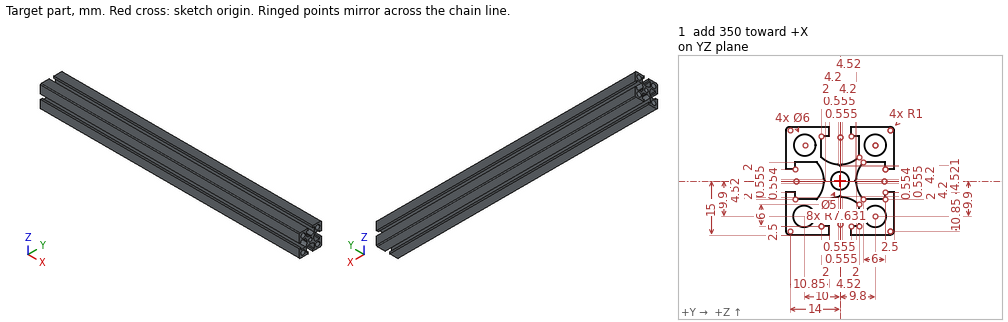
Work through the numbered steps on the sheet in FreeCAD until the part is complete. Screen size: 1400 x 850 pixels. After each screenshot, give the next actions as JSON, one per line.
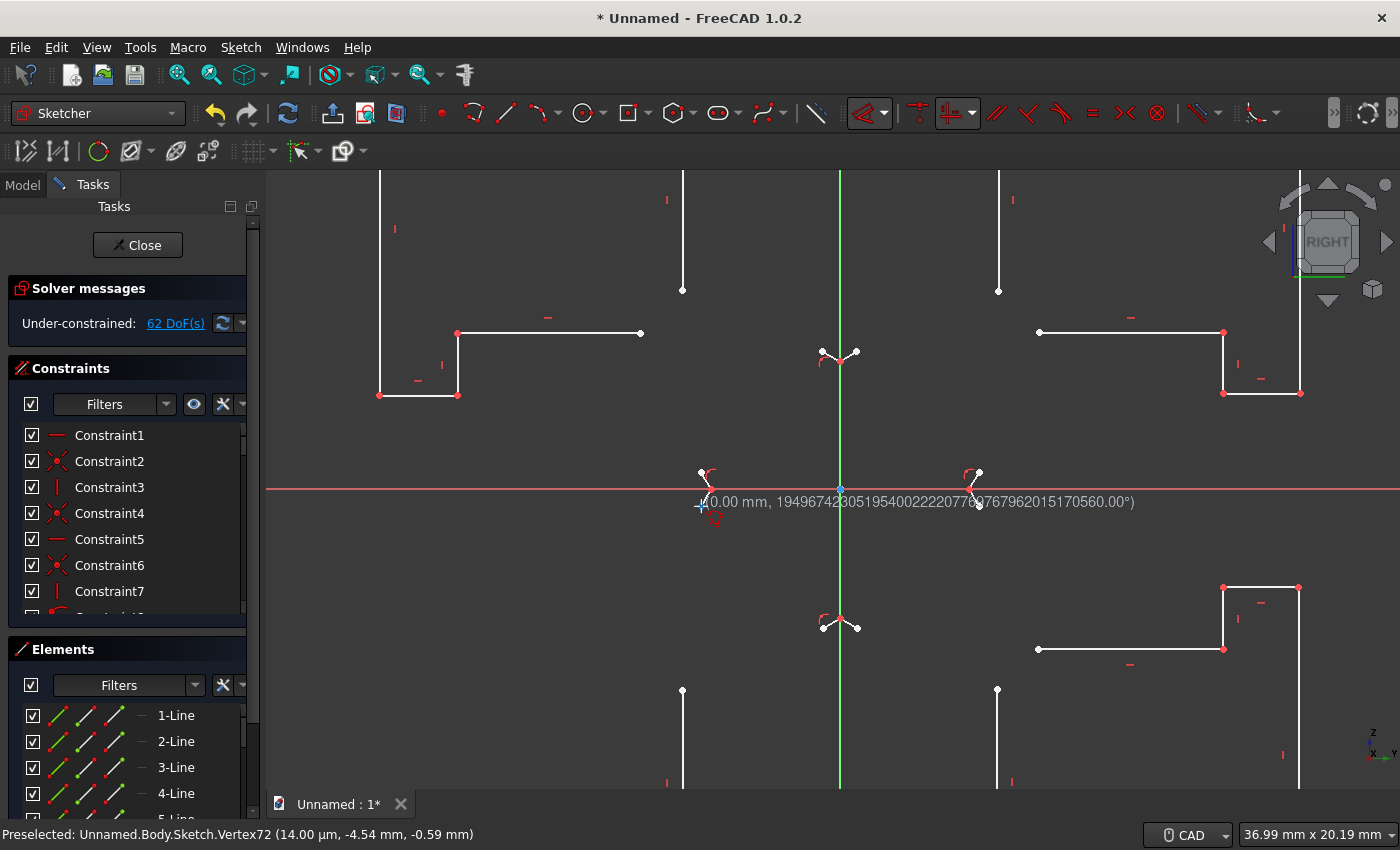
{"action": "left_click", "coordinate": [641, 647]}
{"action": "left_click", "coordinate": [457, 647]}
{"action": "left_click", "coordinate": [457, 586]}
{"action": "left_click", "coordinate": [380, 586]}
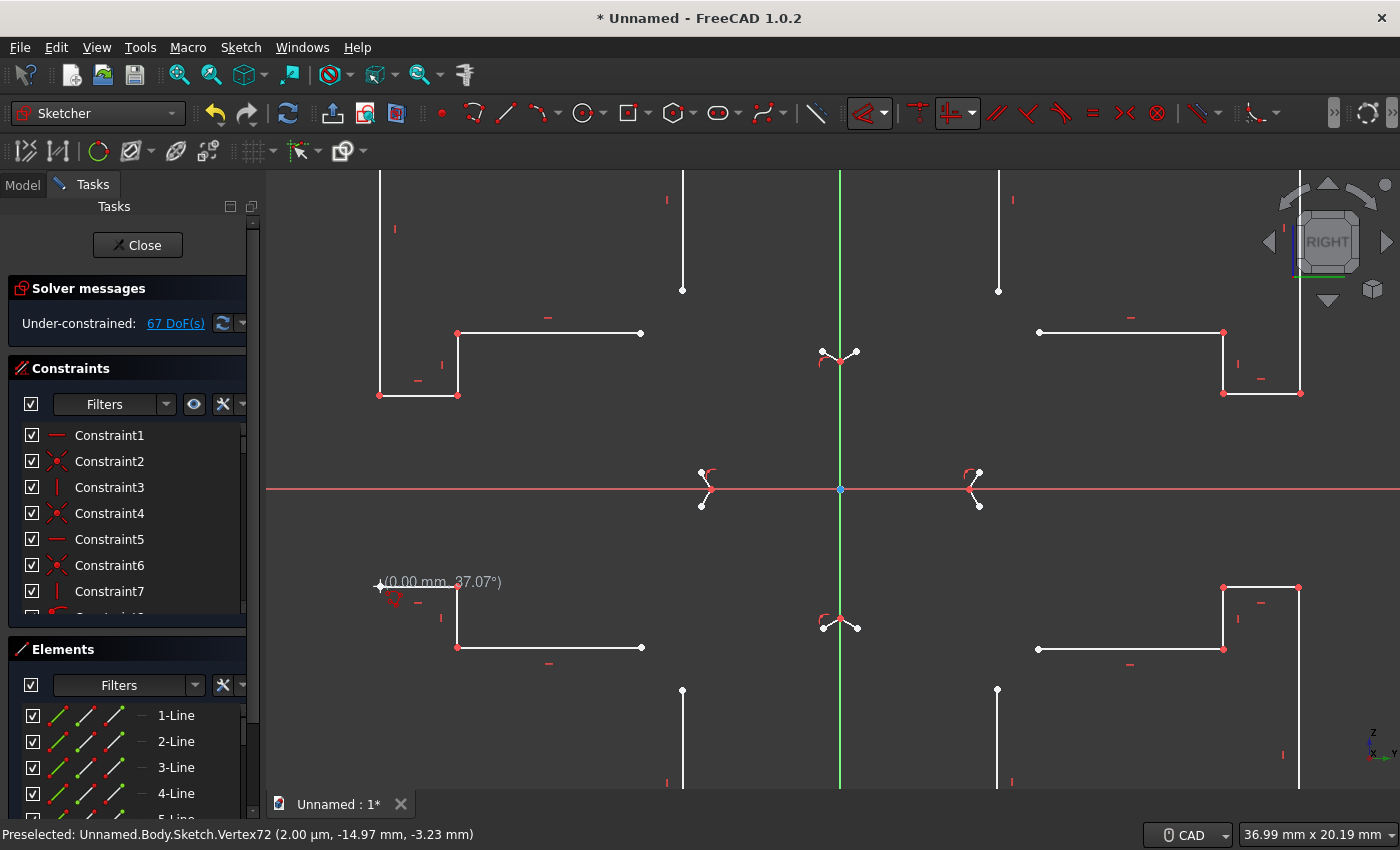
{"action": "scroll", "coordinate": [703, 472], "scroll_direction": "down", "scroll_amount": 4}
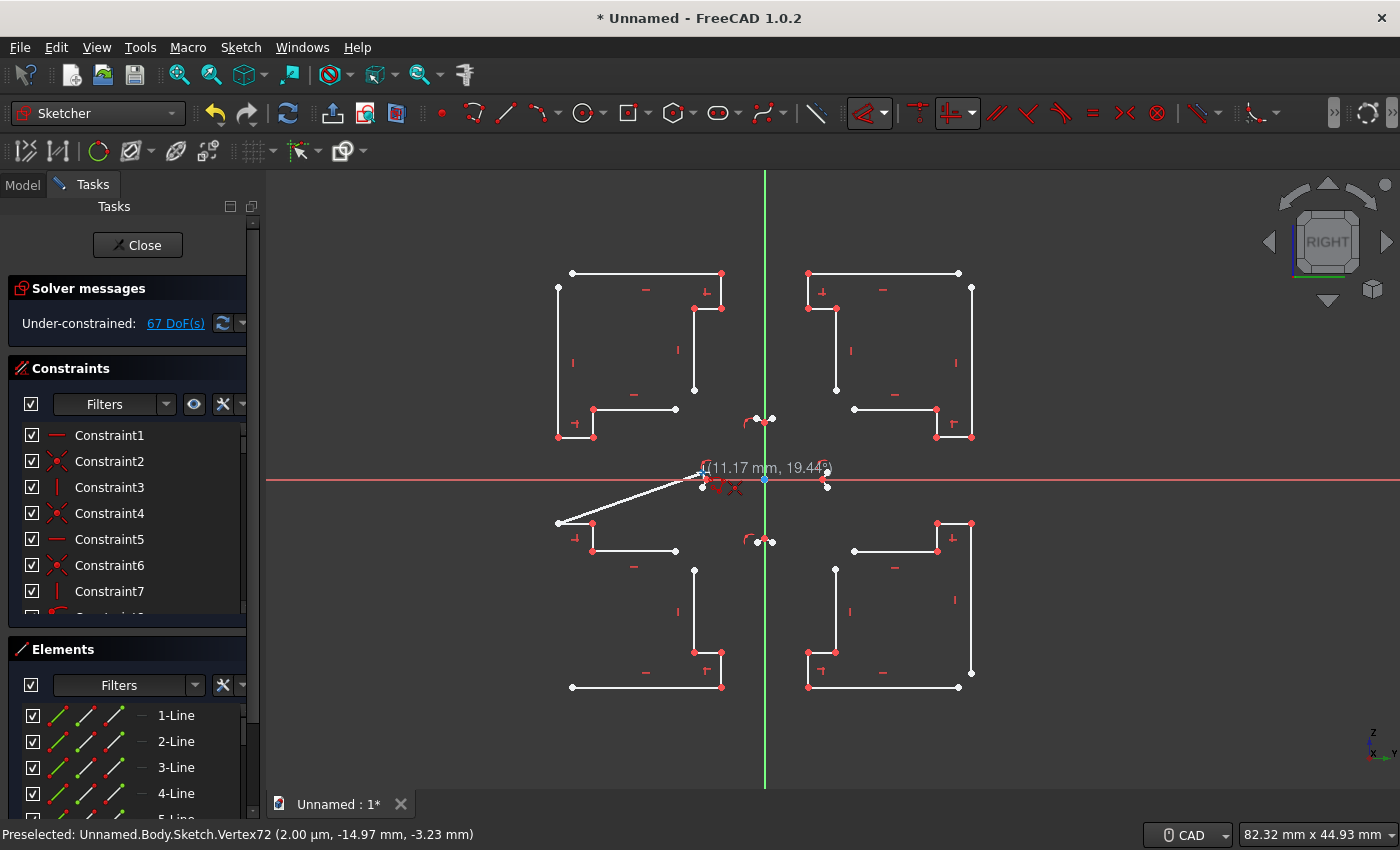
{"action": "left_click", "coordinate": [558, 673]}
{"action": "right_click", "coordinate": [558, 673]}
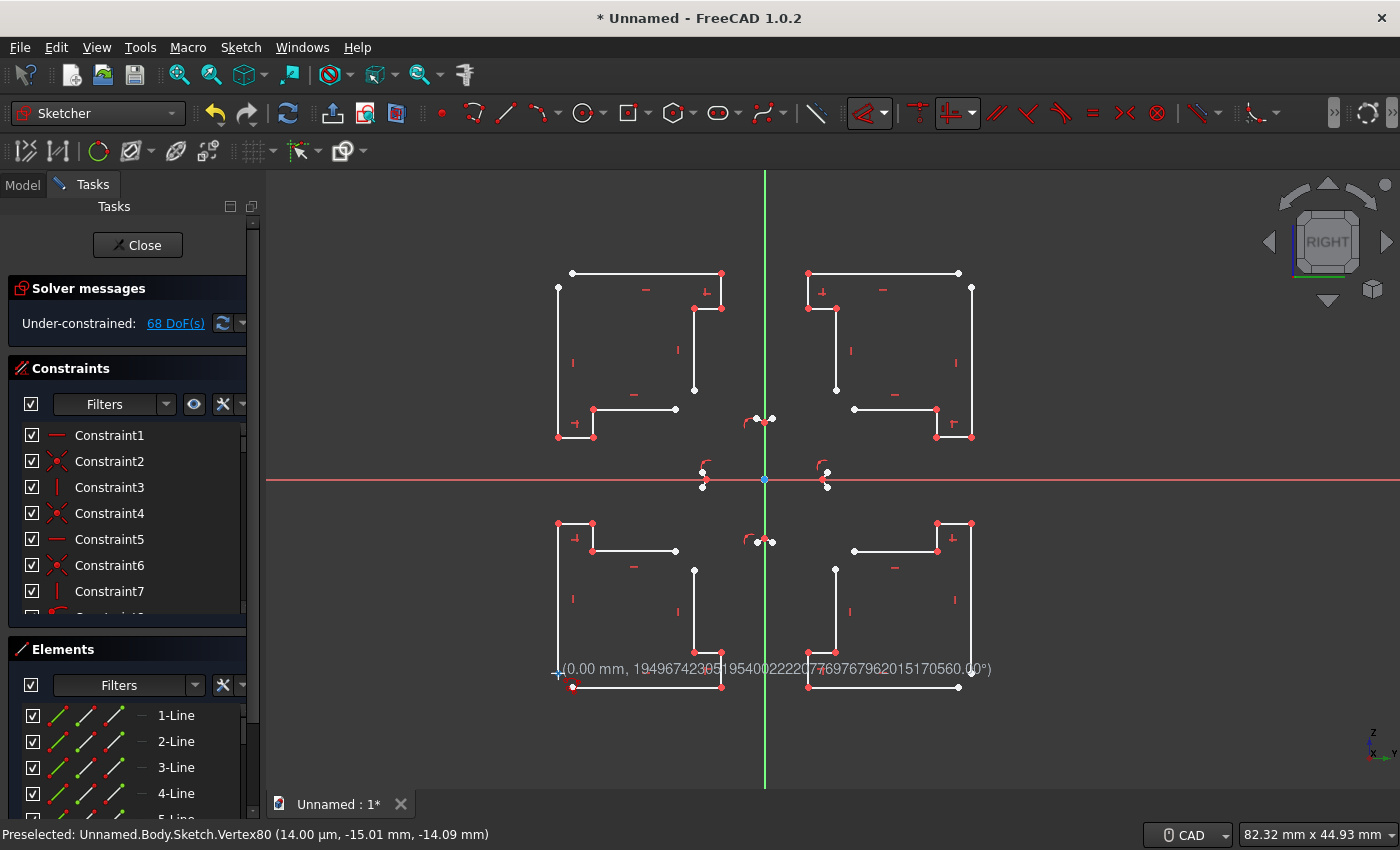
{"action": "left_click", "coordinate": [538, 114]}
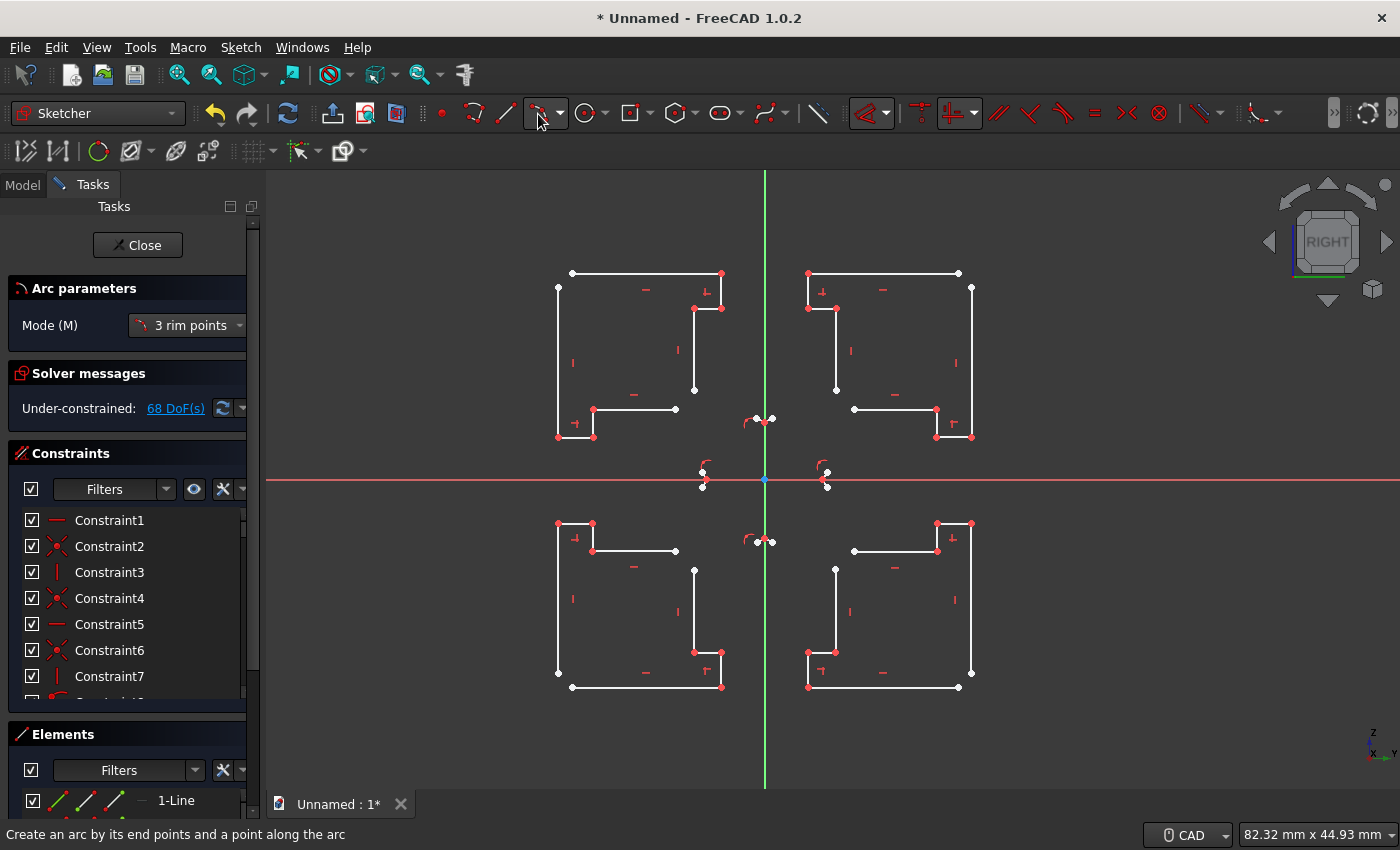
{"action": "left_click", "coordinate": [694, 571]}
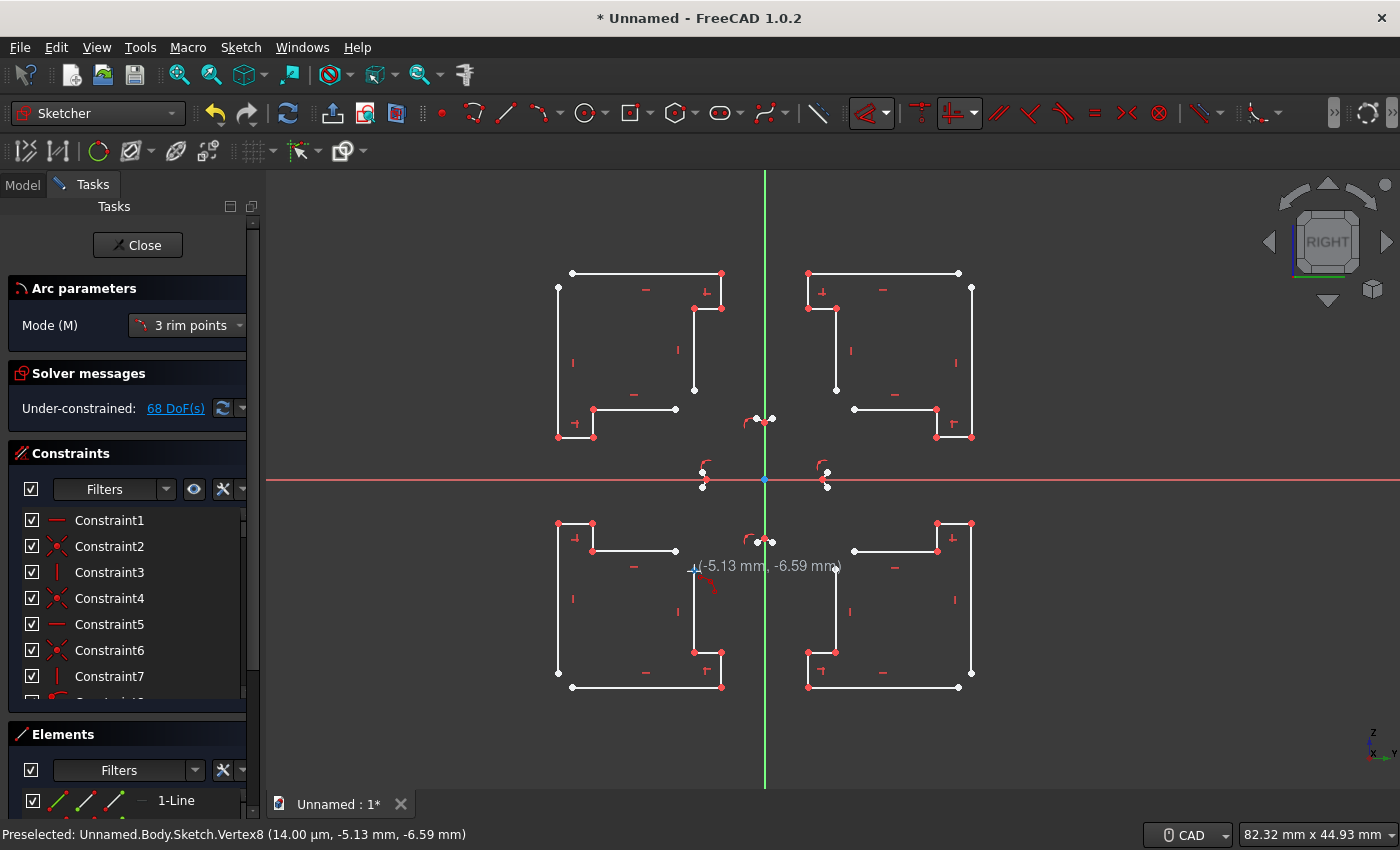
{"action": "scroll", "coordinate": [757, 542], "scroll_direction": "up", "scroll_amount": 7}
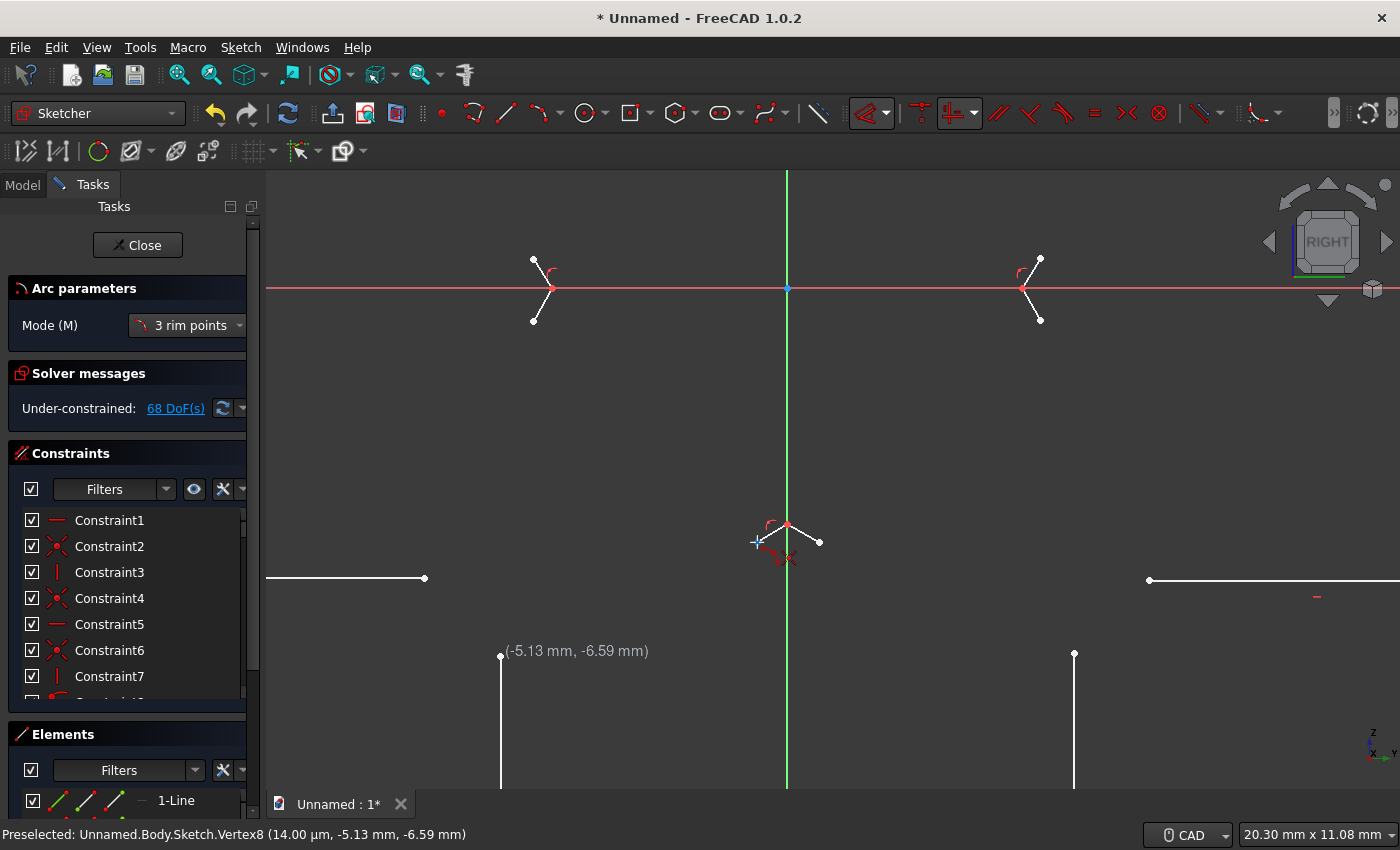
{"action": "left_click", "coordinate": [757, 542]}
{"action": "left_click", "coordinate": [619, 575]}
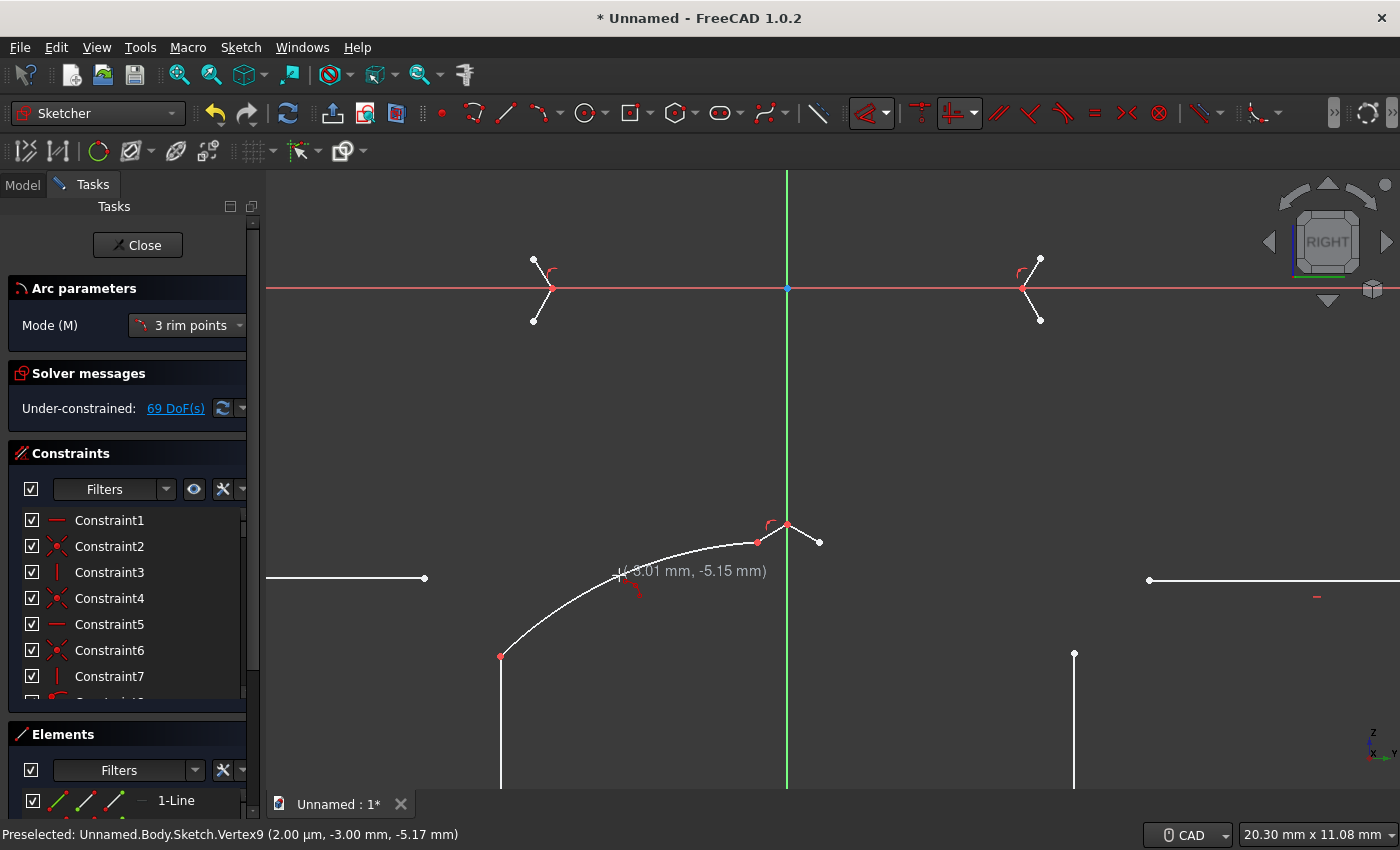
{"action": "left_click", "coordinate": [819, 542]}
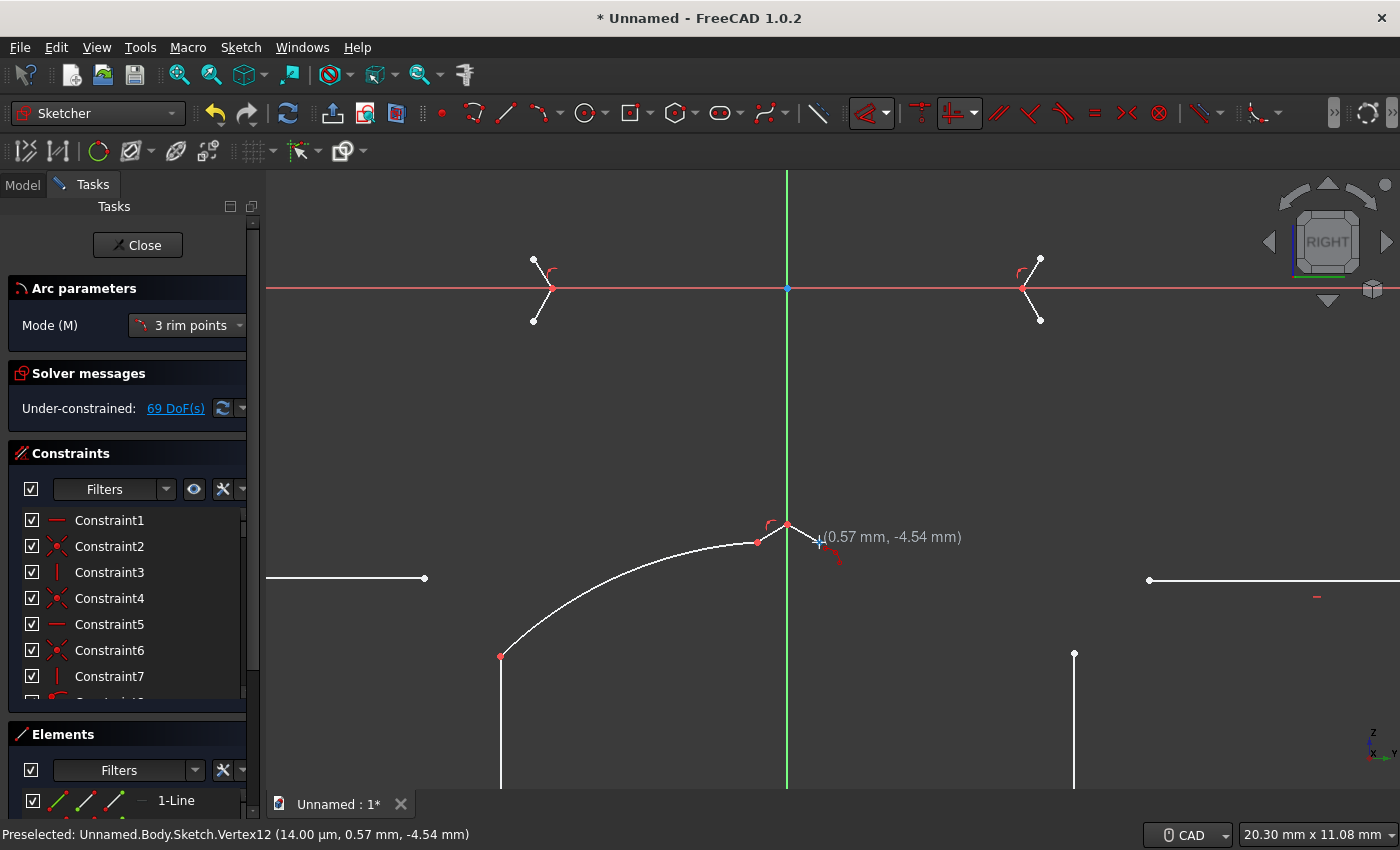
{"action": "scroll", "coordinate": [757, 542], "scroll_direction": "down", "scroll_amount": 7}